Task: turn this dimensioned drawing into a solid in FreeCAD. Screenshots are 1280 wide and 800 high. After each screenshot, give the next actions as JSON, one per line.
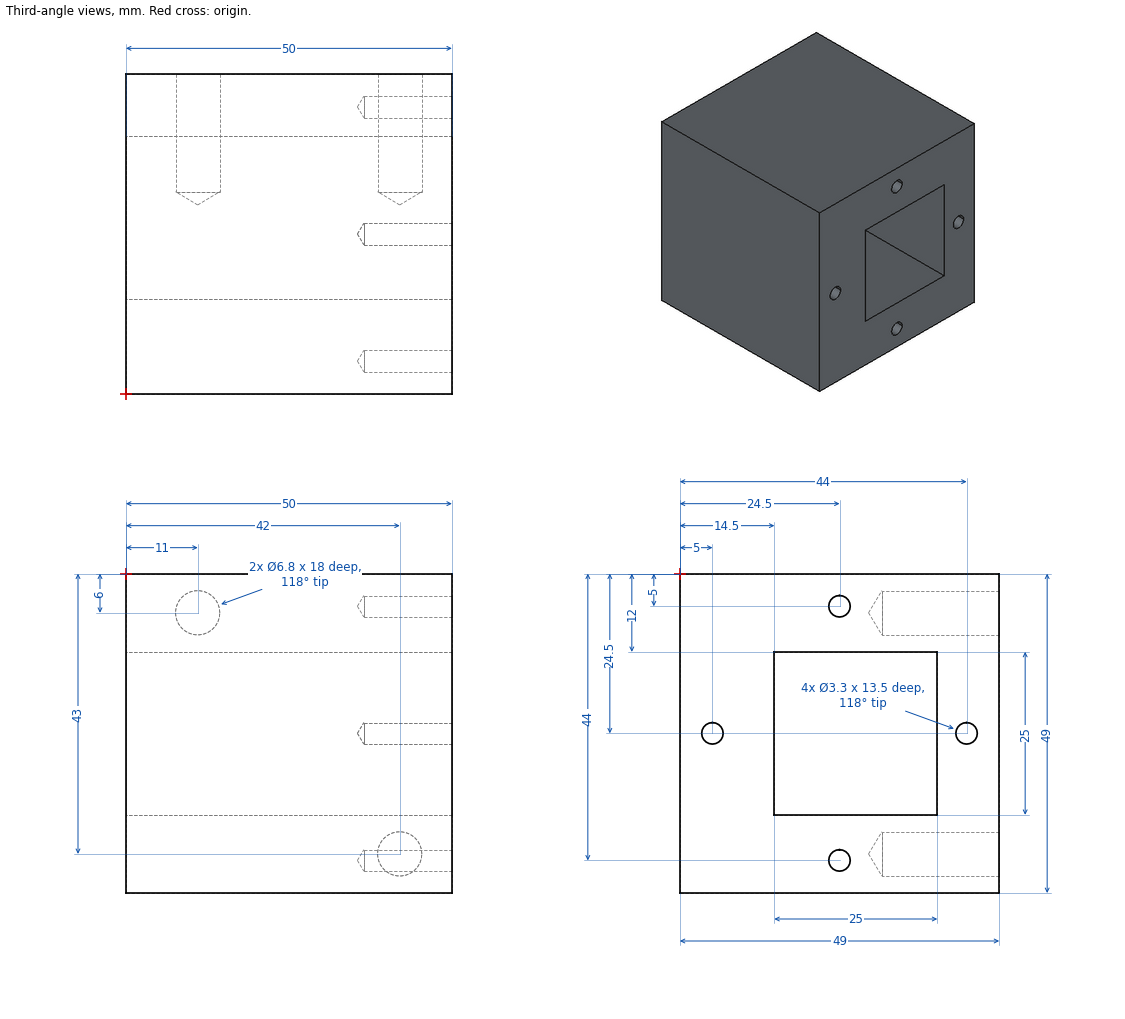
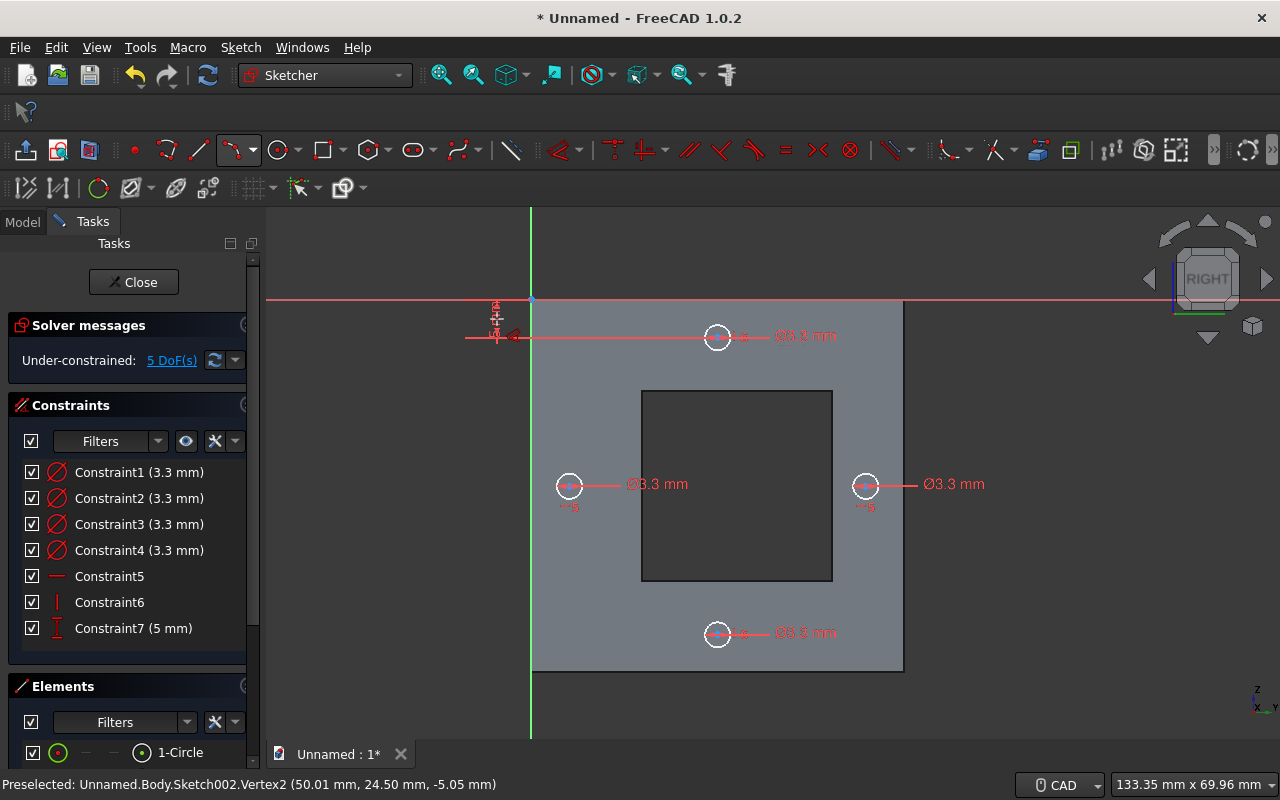
{"action": "left_click", "coordinate": [569, 486]}
{"action": "left_click", "coordinate": [550, 266]}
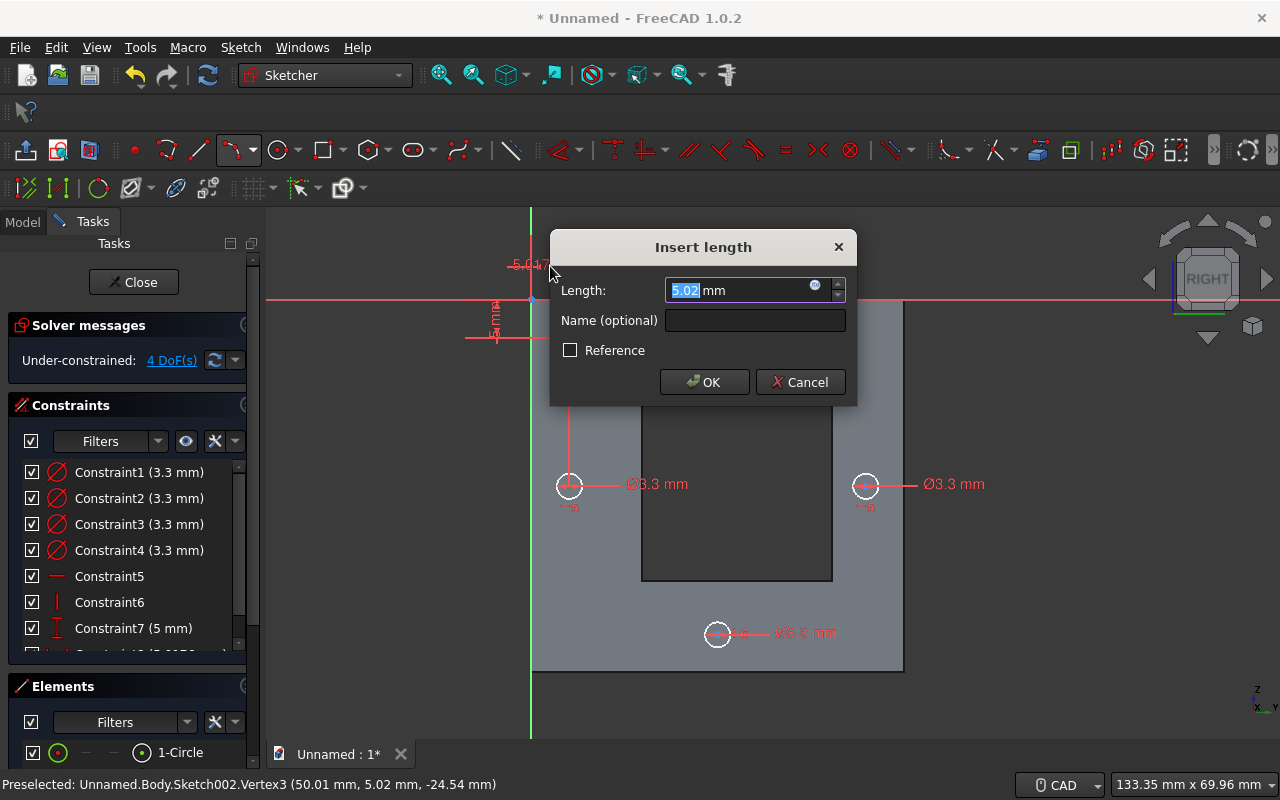
{"action": "type", "text": "5"}
{"action": "key", "text": "Return"}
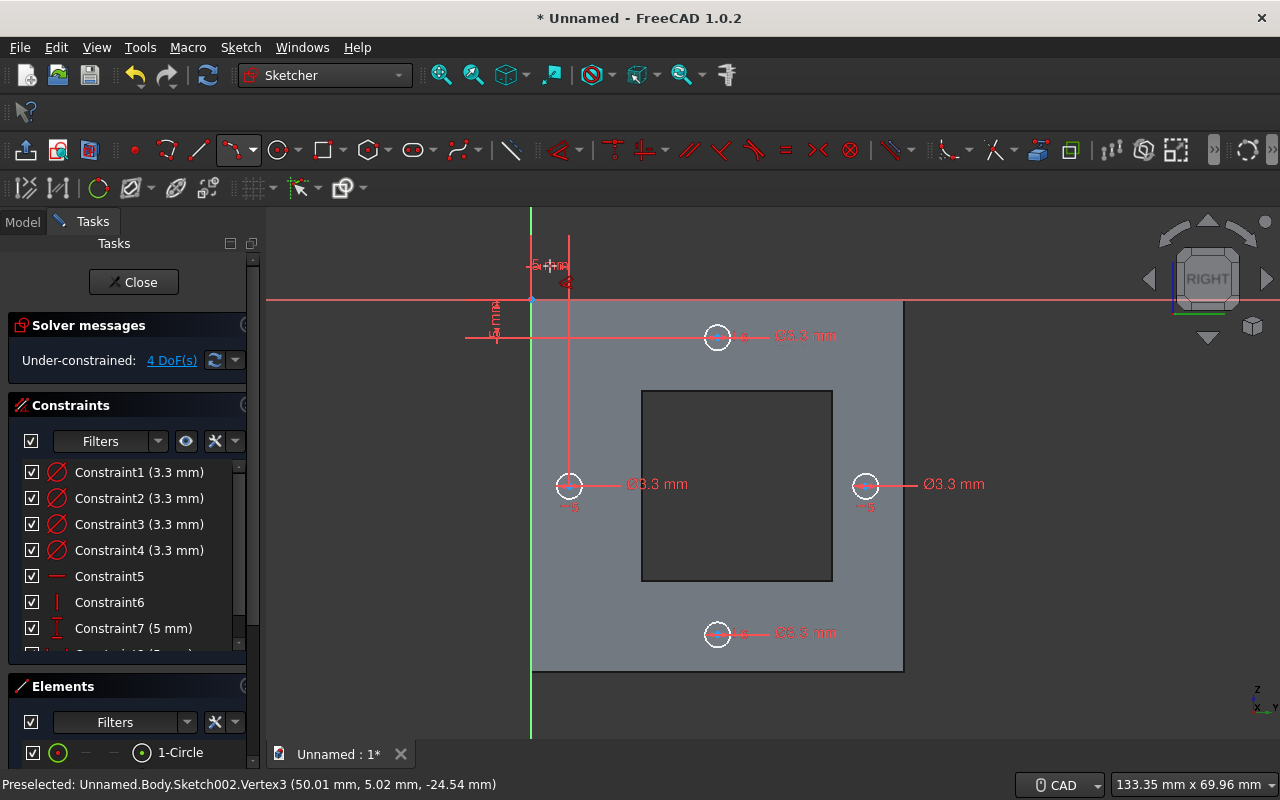
{"action": "left_click", "coordinate": [866, 486]}
{"action": "left_click", "coordinate": [699, 266]}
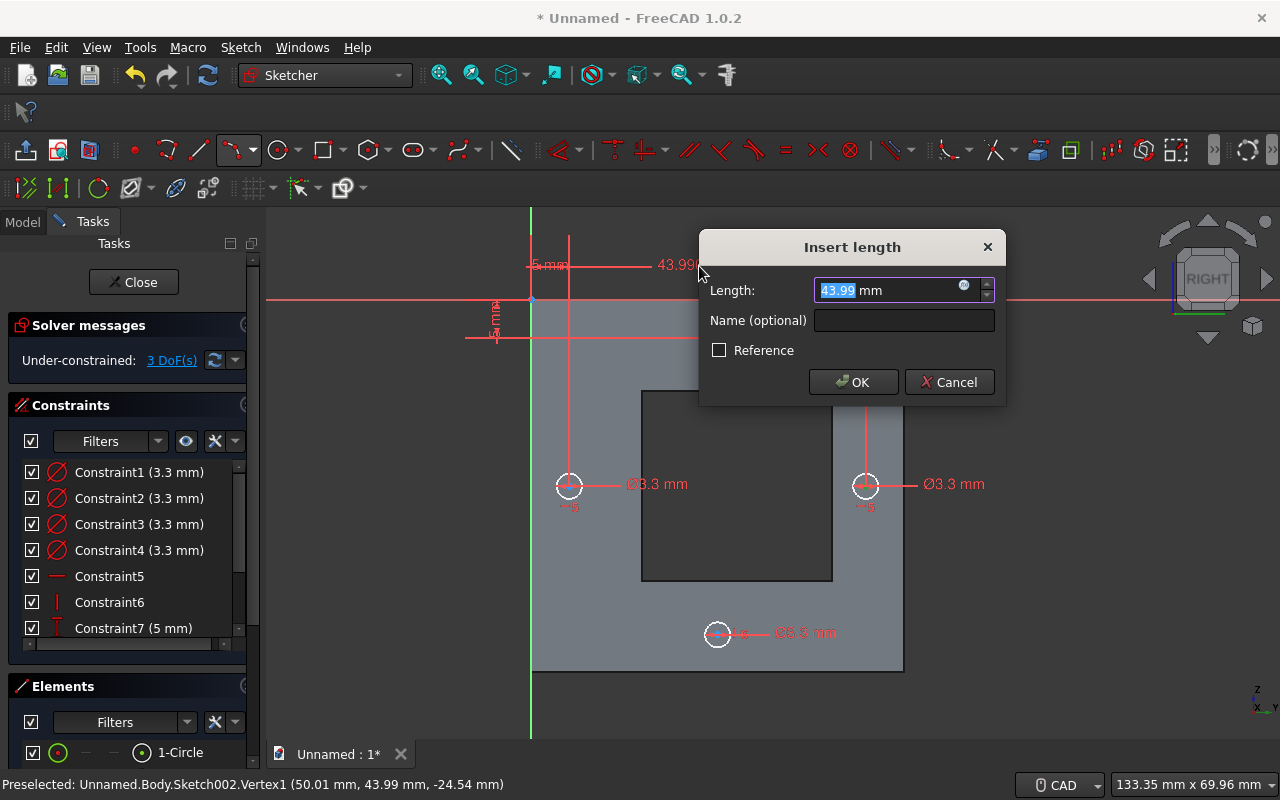
{"action": "type", "text": "44"}
{"action": "key", "text": "Return"}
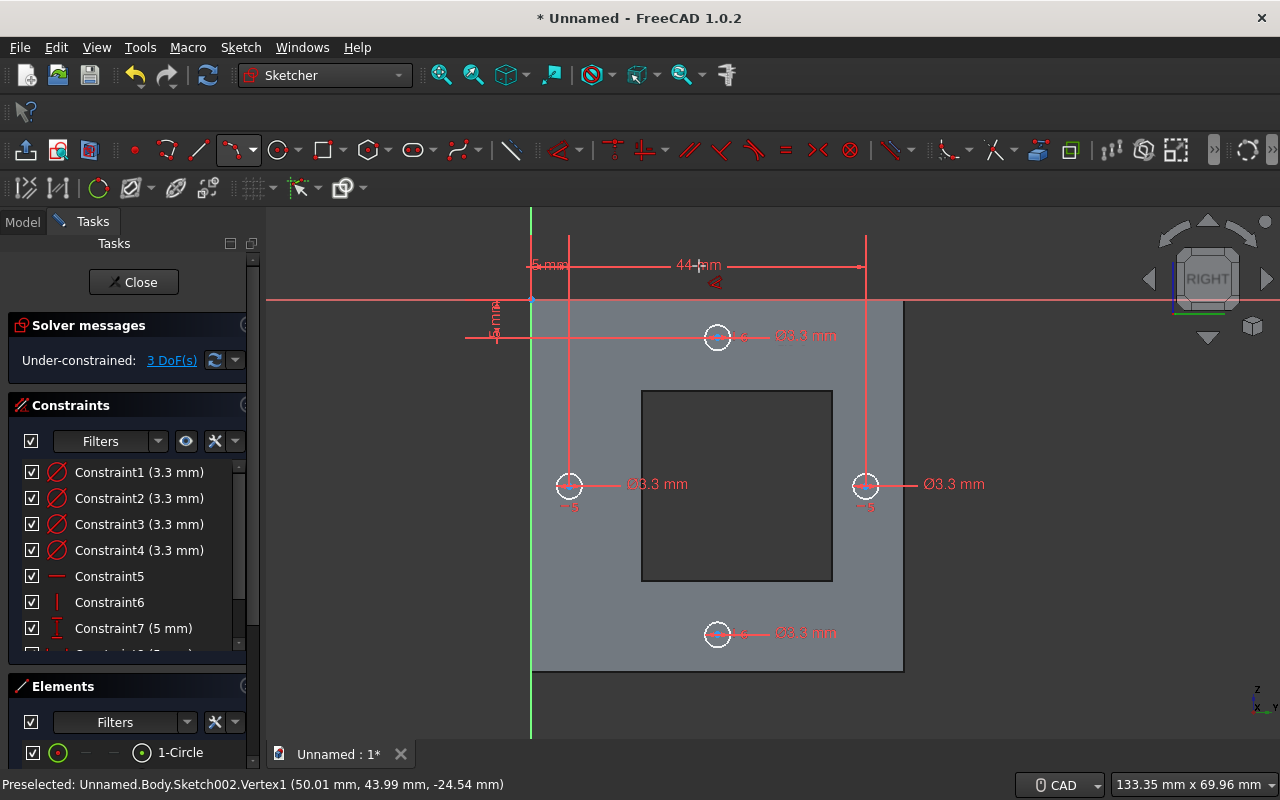
{"action": "left_click", "coordinate": [718, 635]}
{"action": "left_click", "coordinate": [497, 467]}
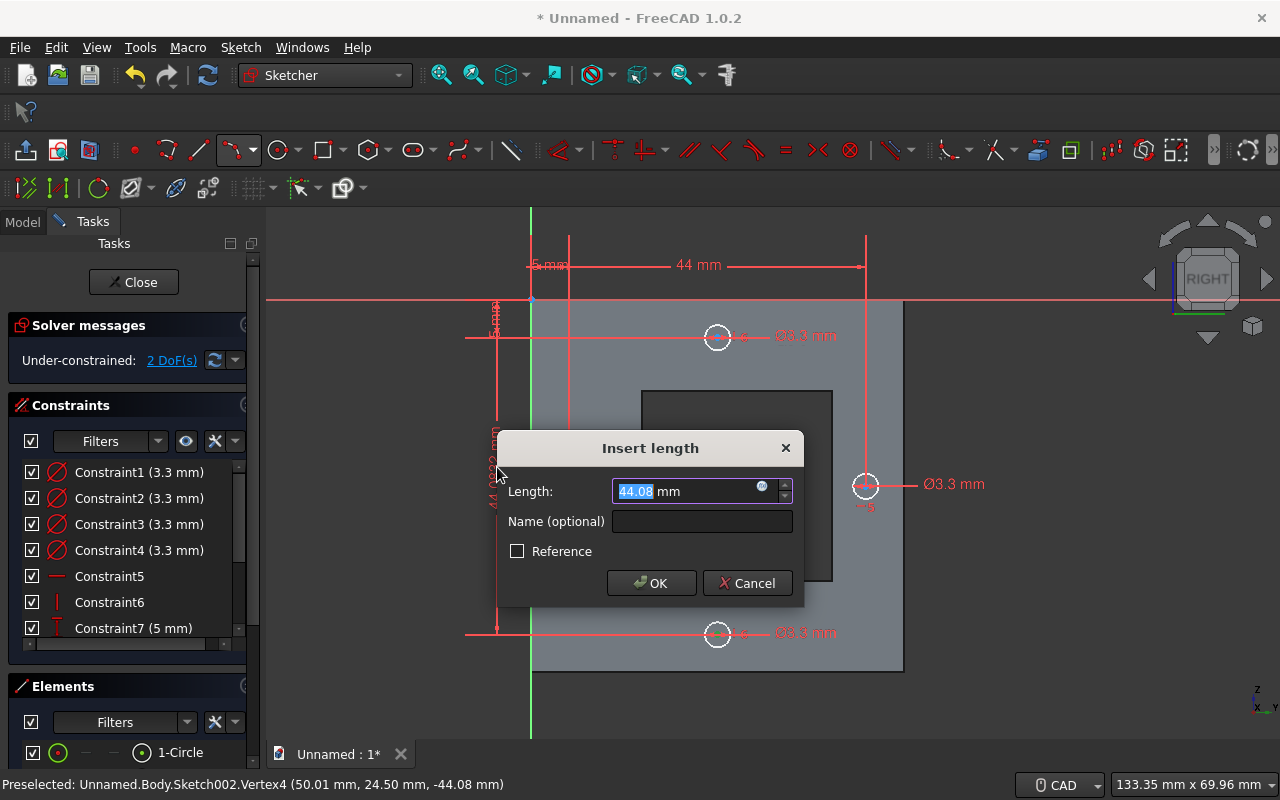
{"action": "type", "text": "44"}
{"action": "key", "text": "Return"}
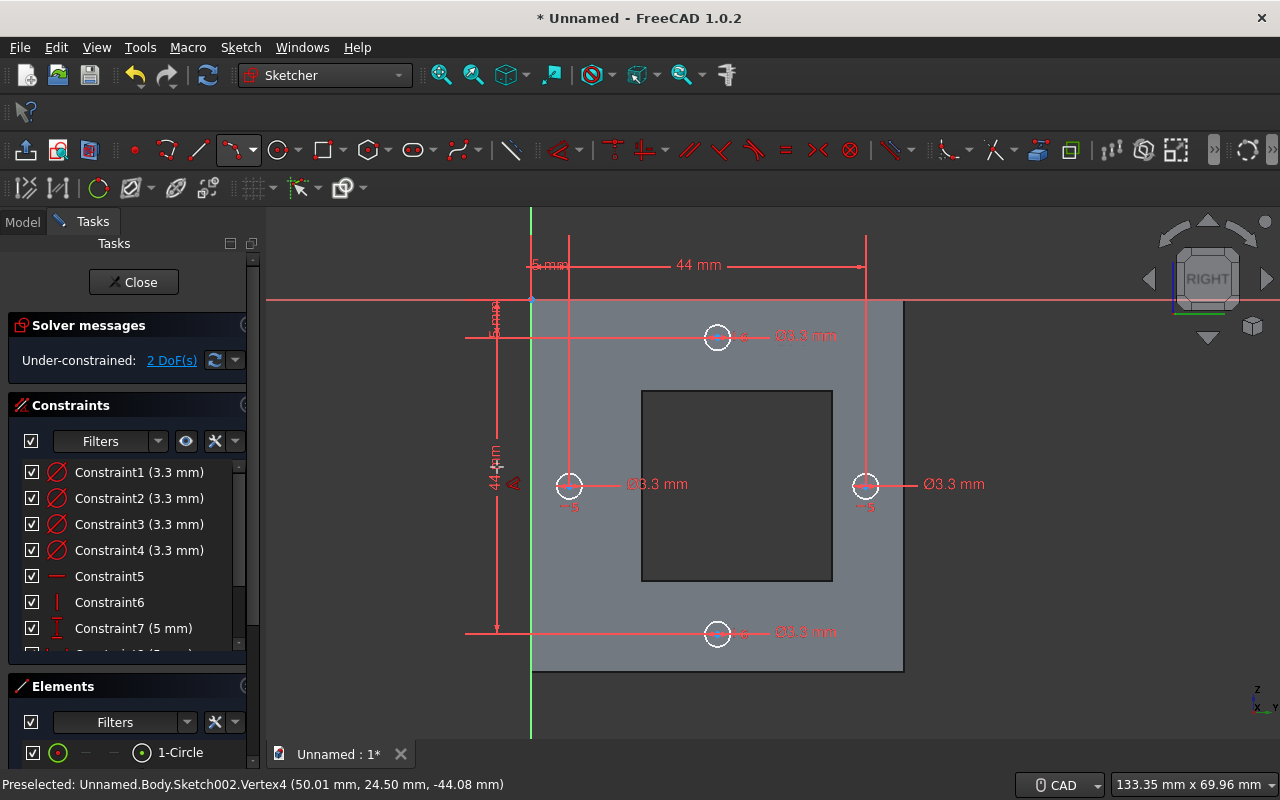
{"action": "left_click", "coordinate": [866, 486]}
{"action": "left_click", "coordinate": [497, 393]}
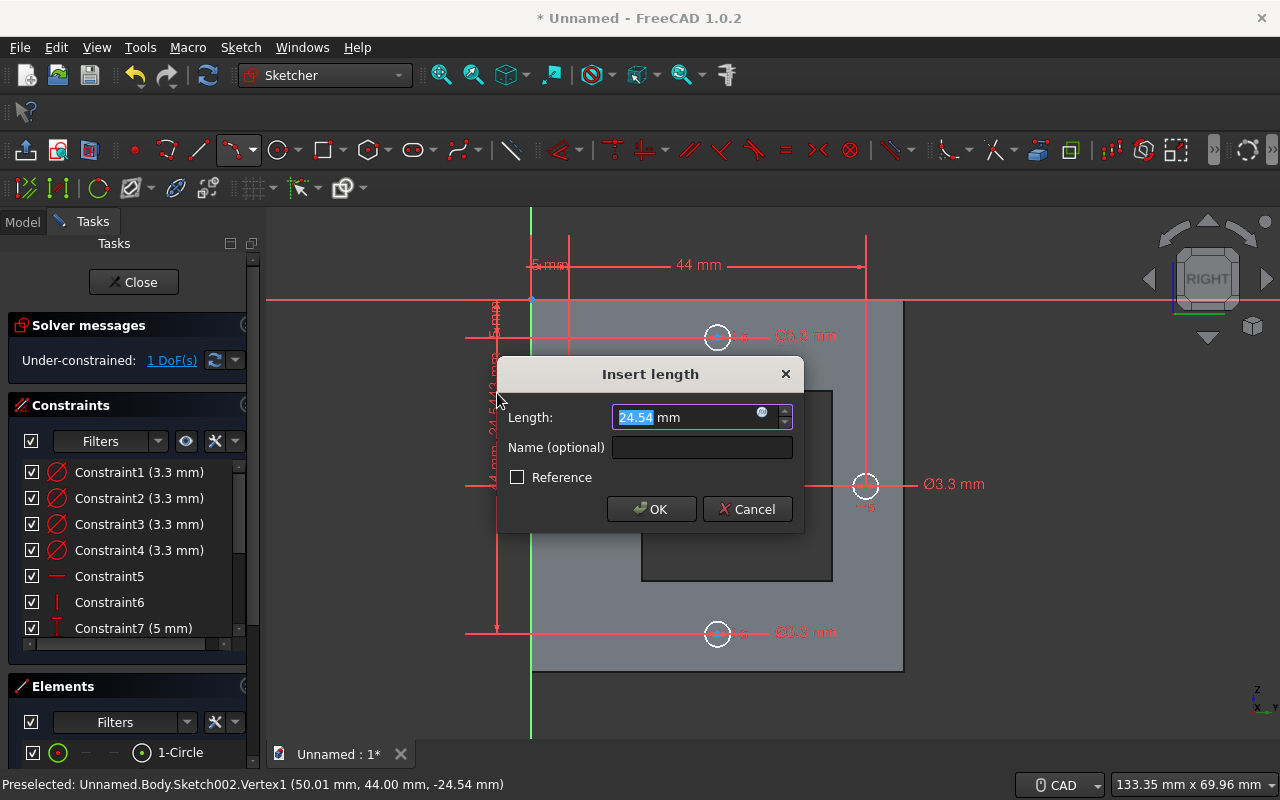
{"action": "type", "text": "24.5"}
{"action": "key", "text": "Return"}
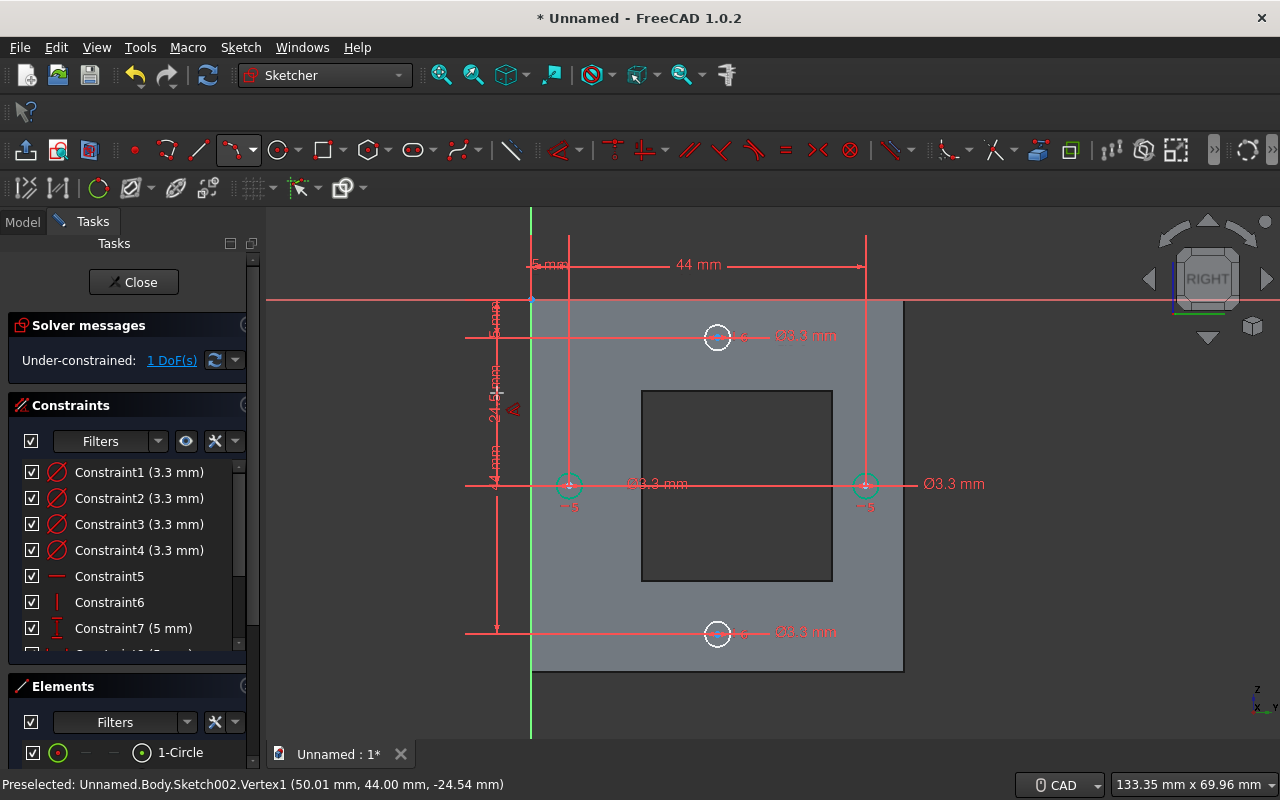
{"action": "left_click", "coordinate": [718, 338]}
{"action": "left_click", "coordinate": [624, 266]}